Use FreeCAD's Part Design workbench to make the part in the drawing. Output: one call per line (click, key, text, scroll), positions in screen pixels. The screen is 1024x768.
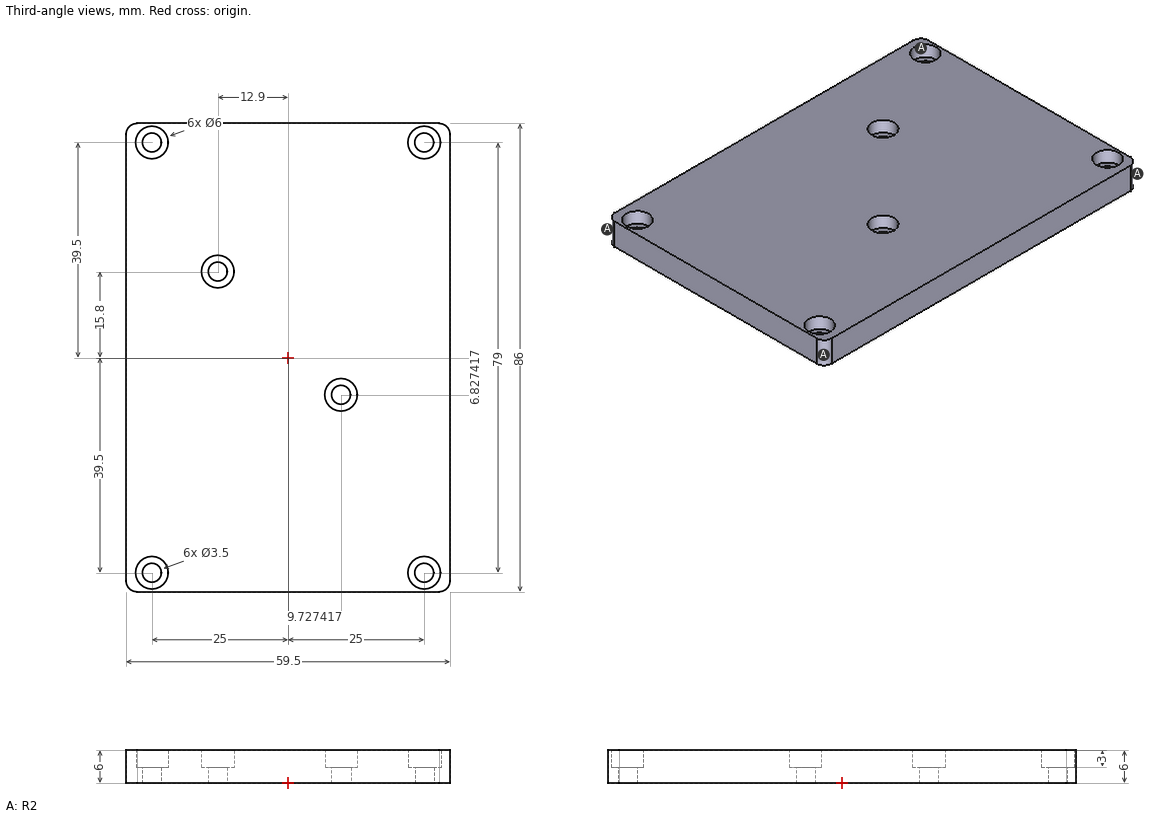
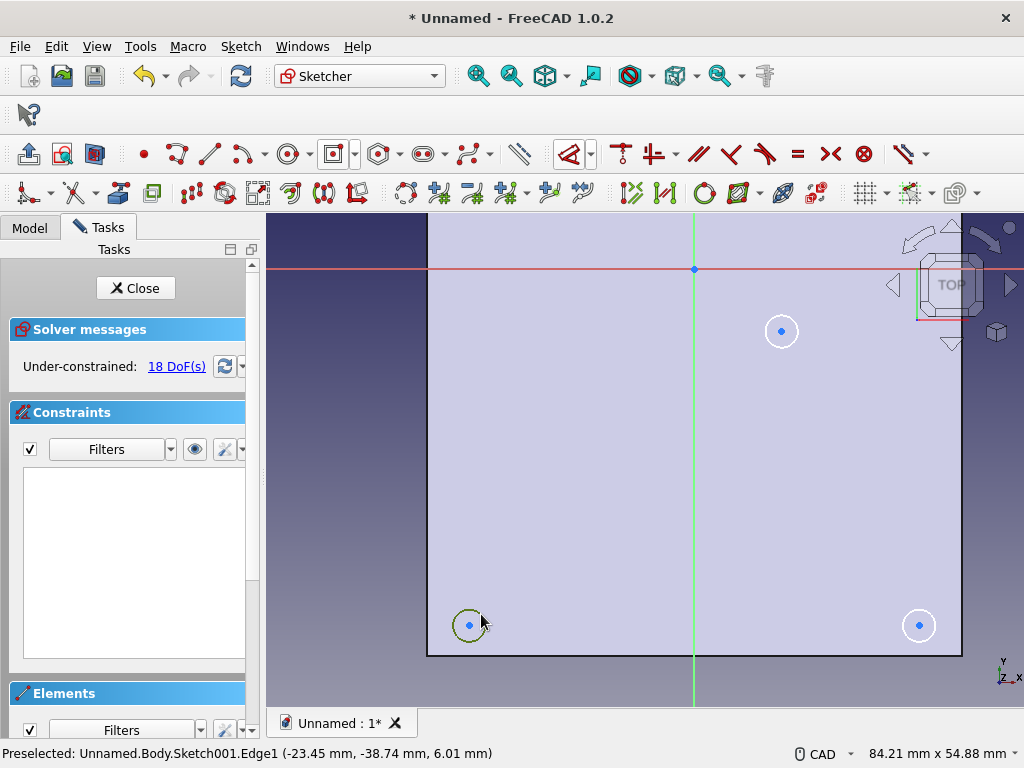
scroll(480, 616, down, 4)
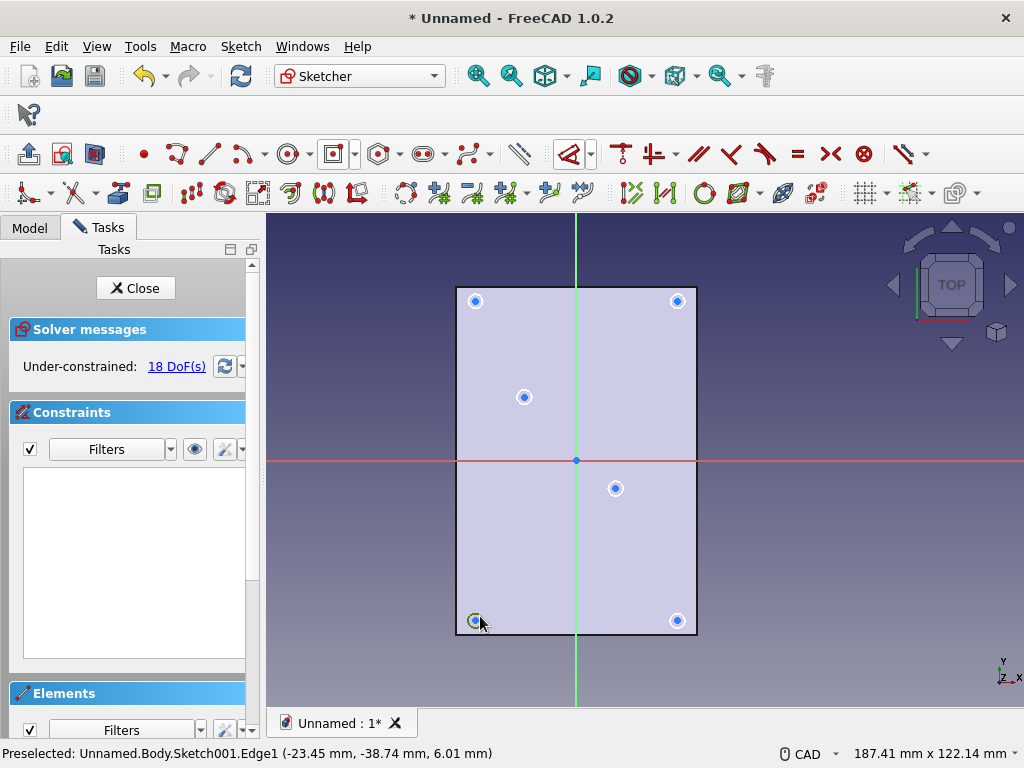
scroll(683, 616, up, 4)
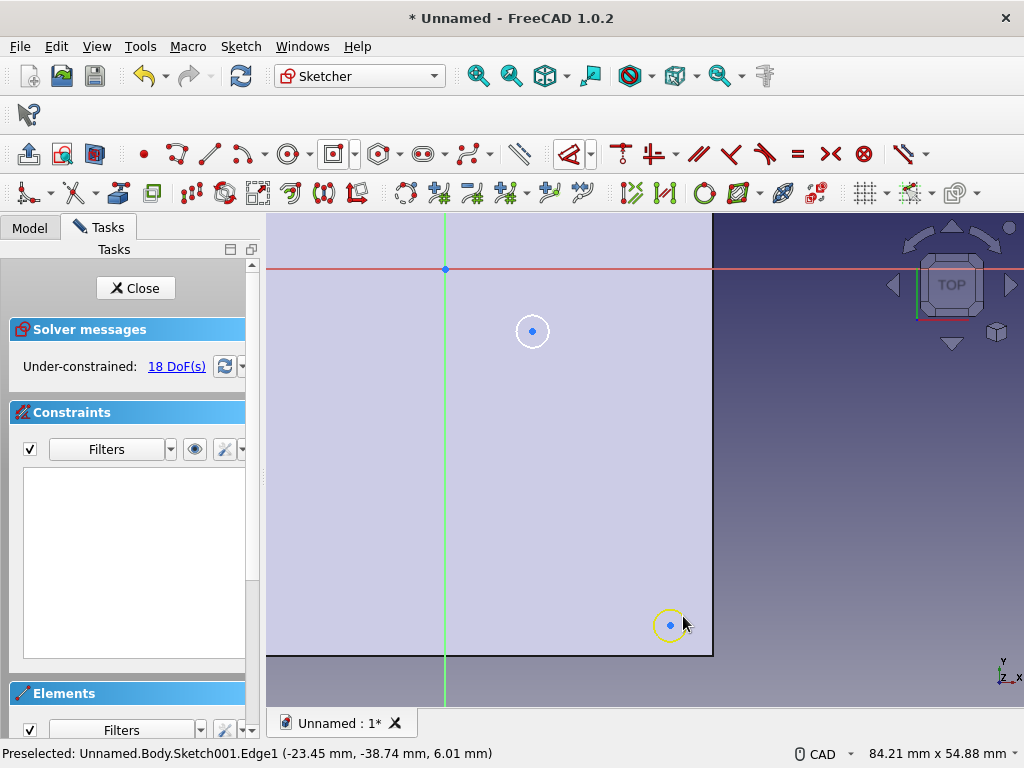
click(681, 614)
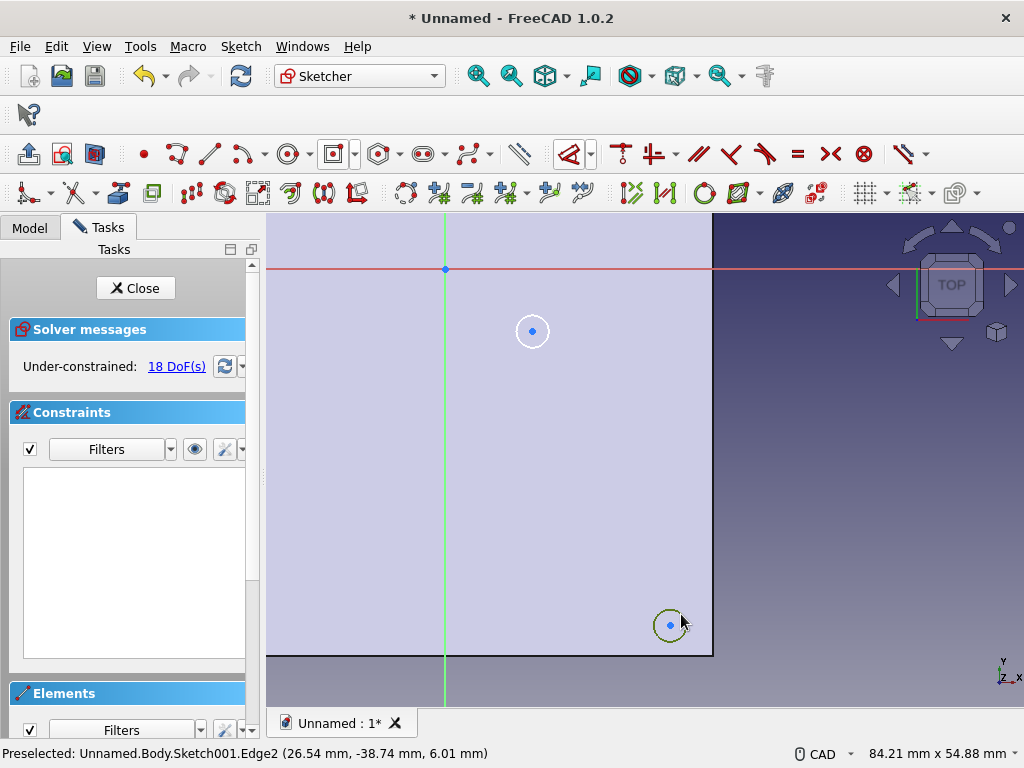
scroll(684, 616, down, 4)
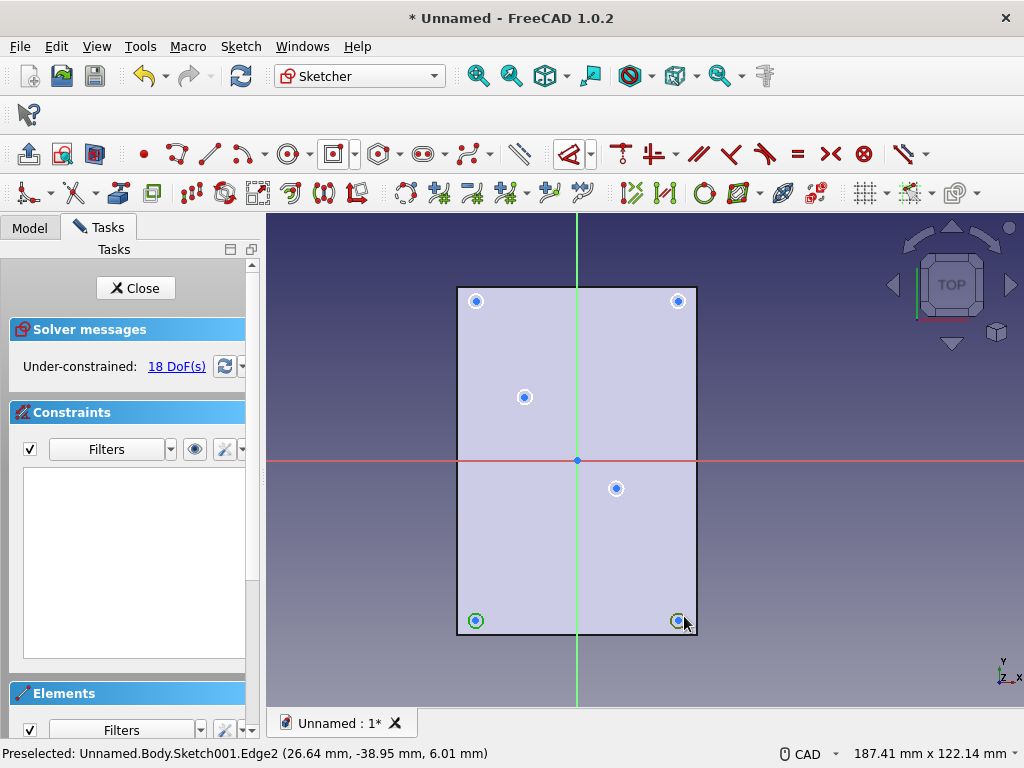
scroll(683, 296, up, 4)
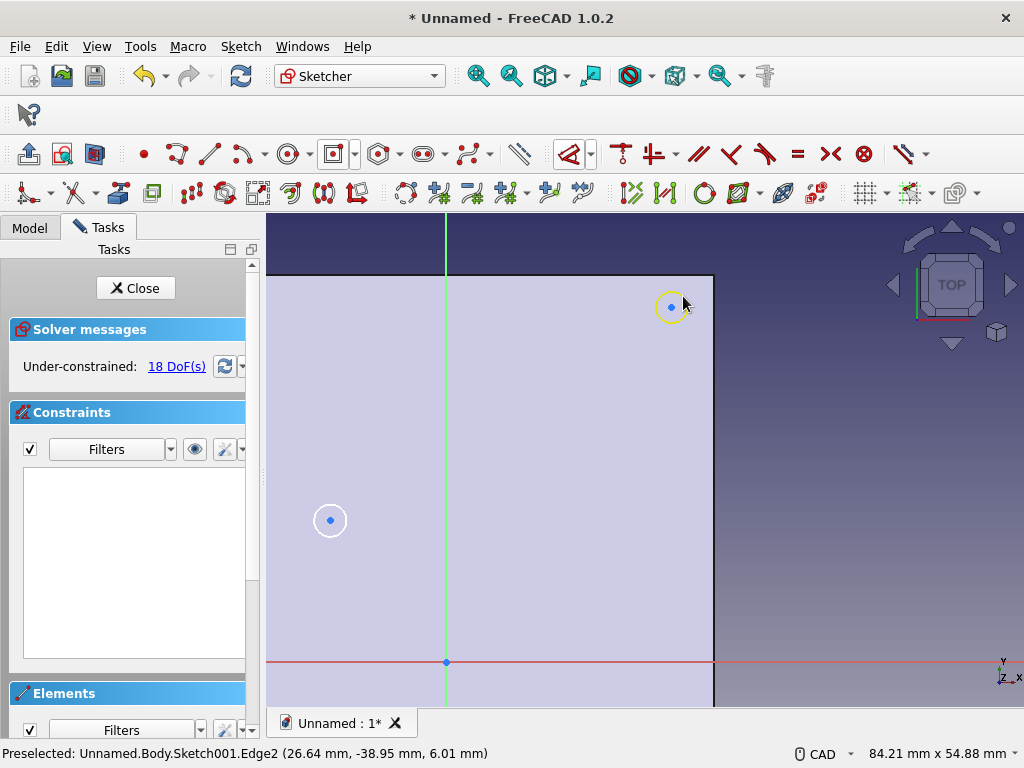
click(683, 296)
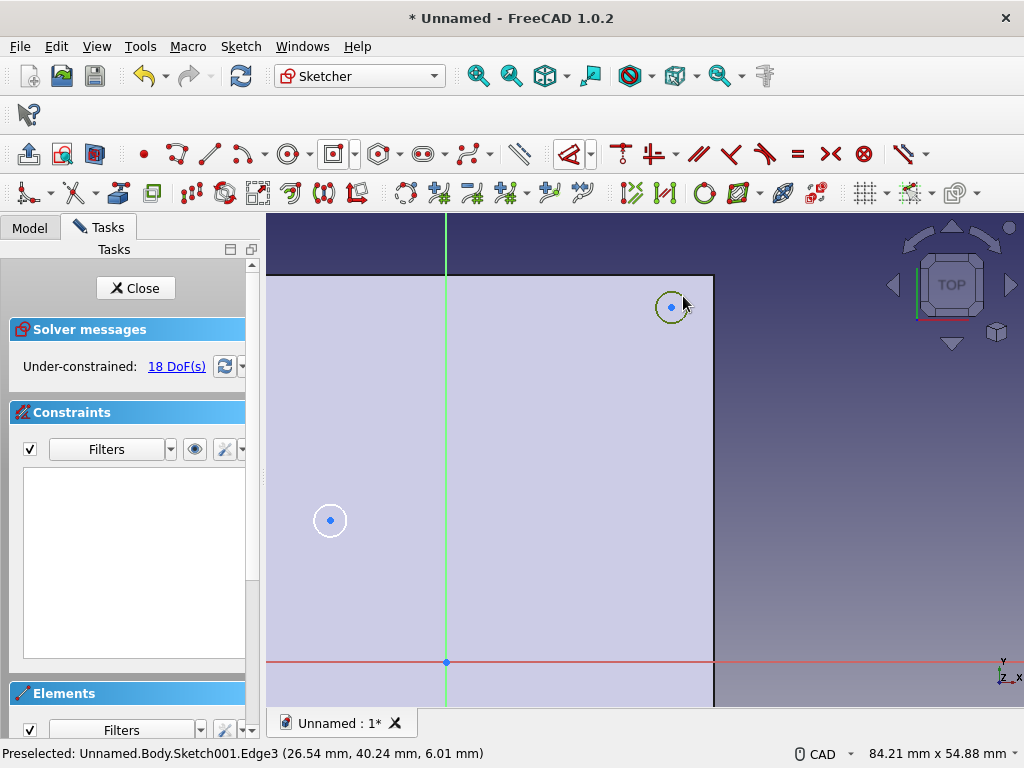
scroll(683, 295, down, 4)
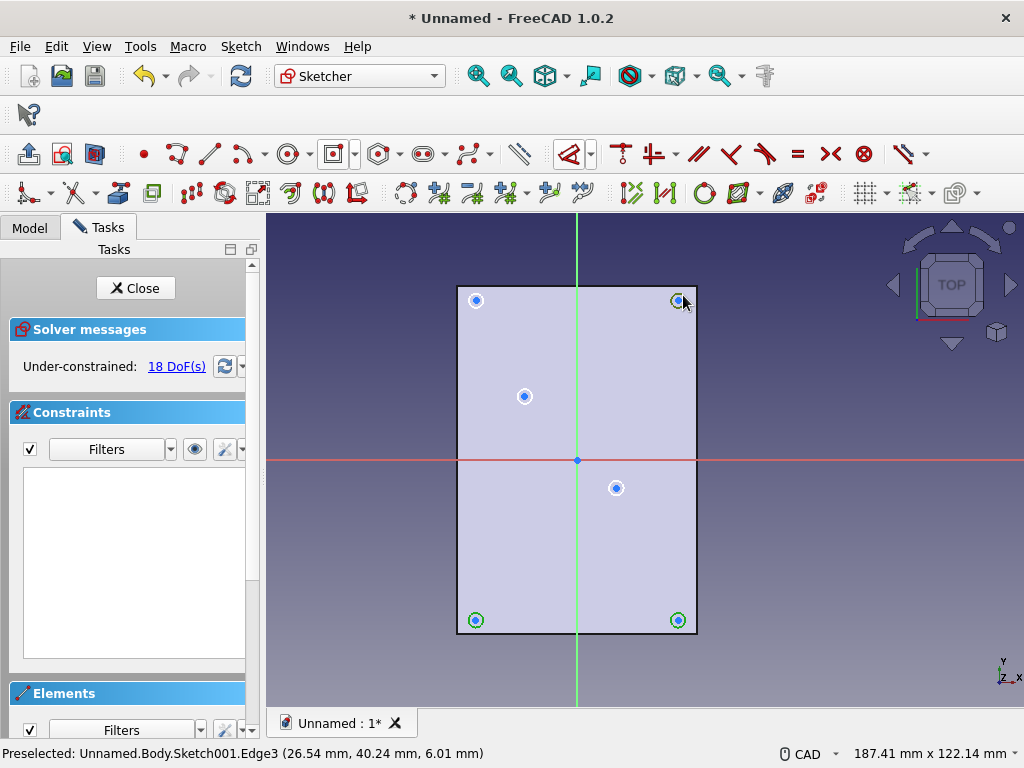
scroll(481, 296, up, 4)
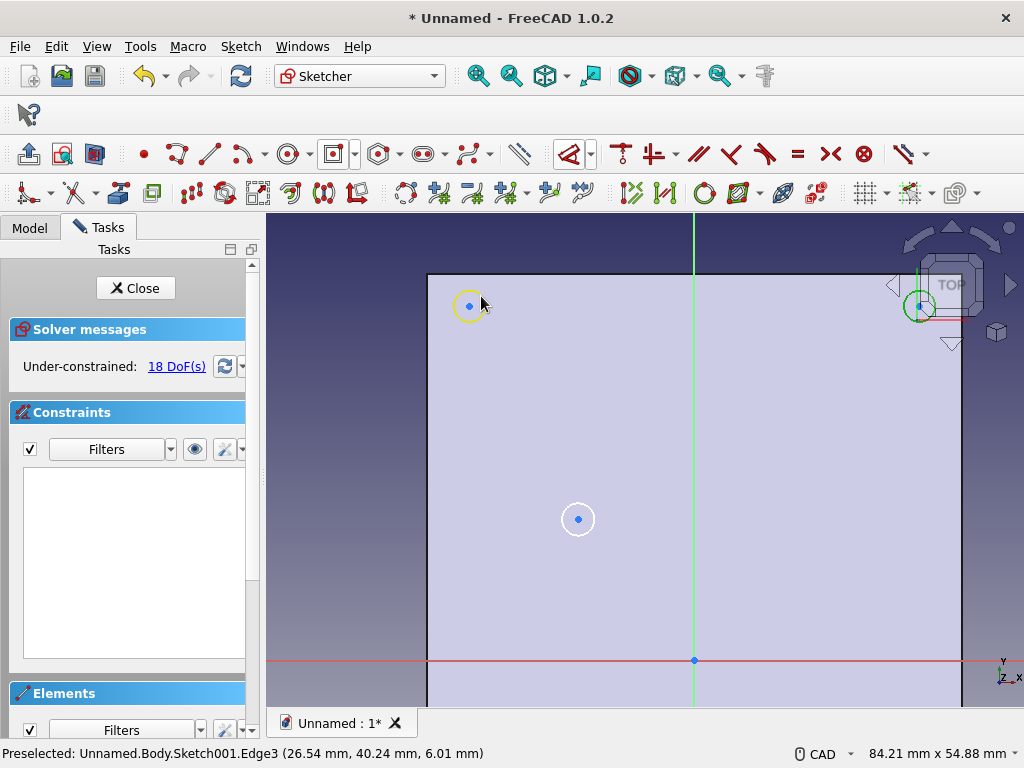
click(481, 295)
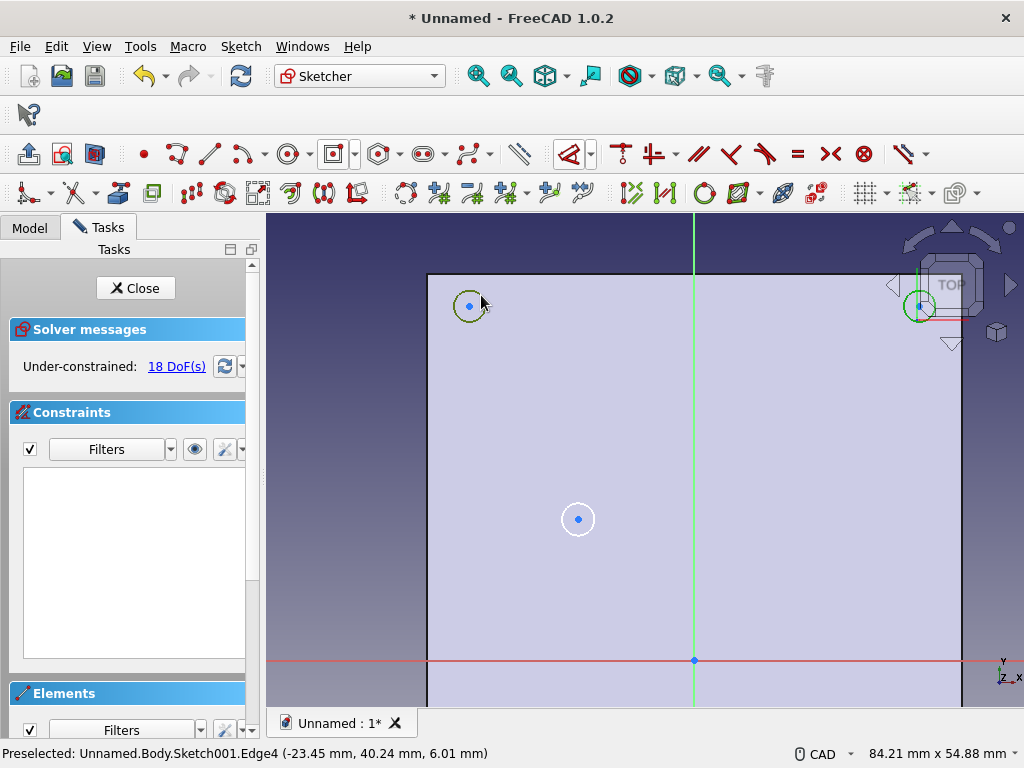
click(590, 508)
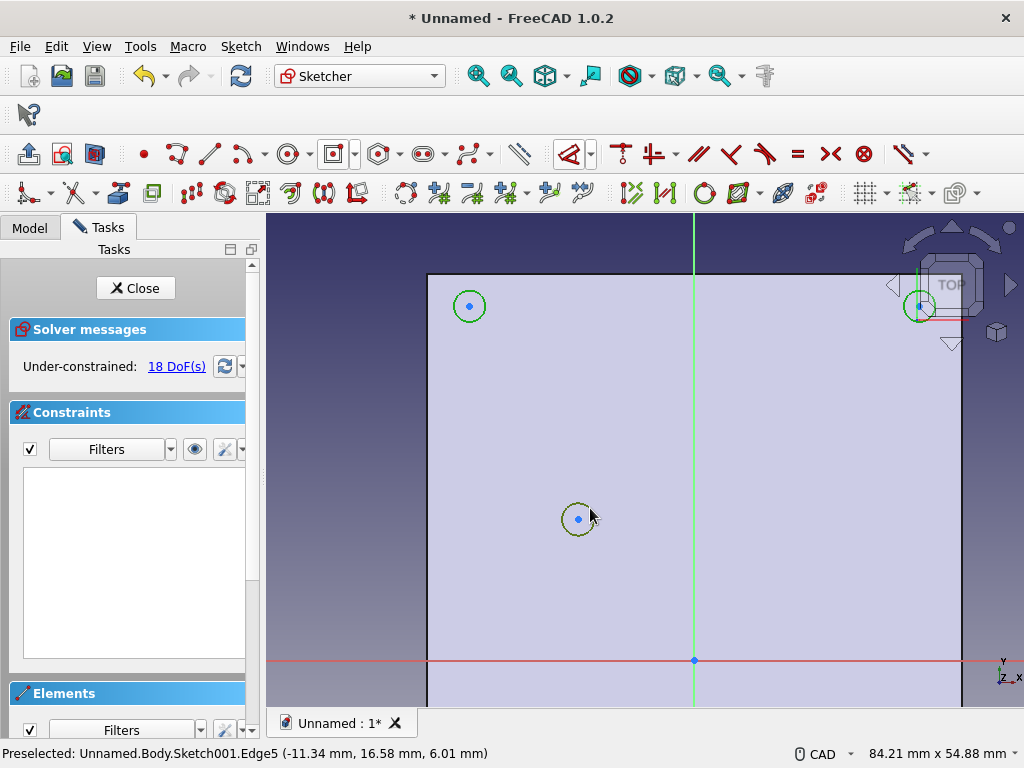
scroll(480, 296, down, 4)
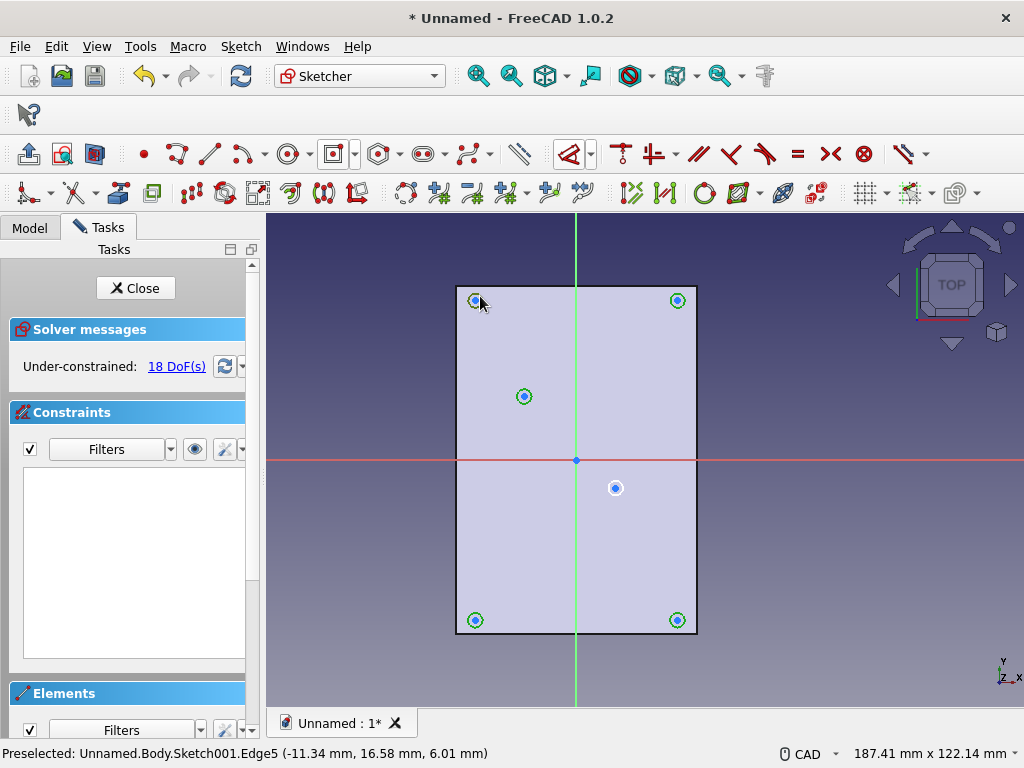
scroll(621, 483, up, 4)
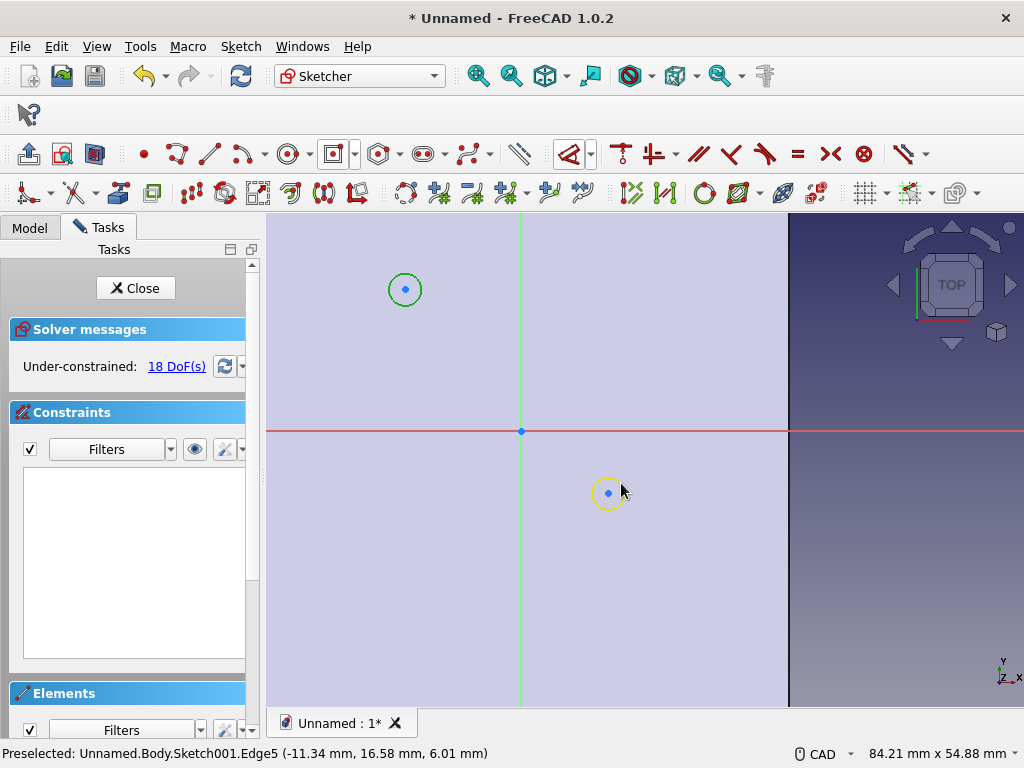
click(620, 482)